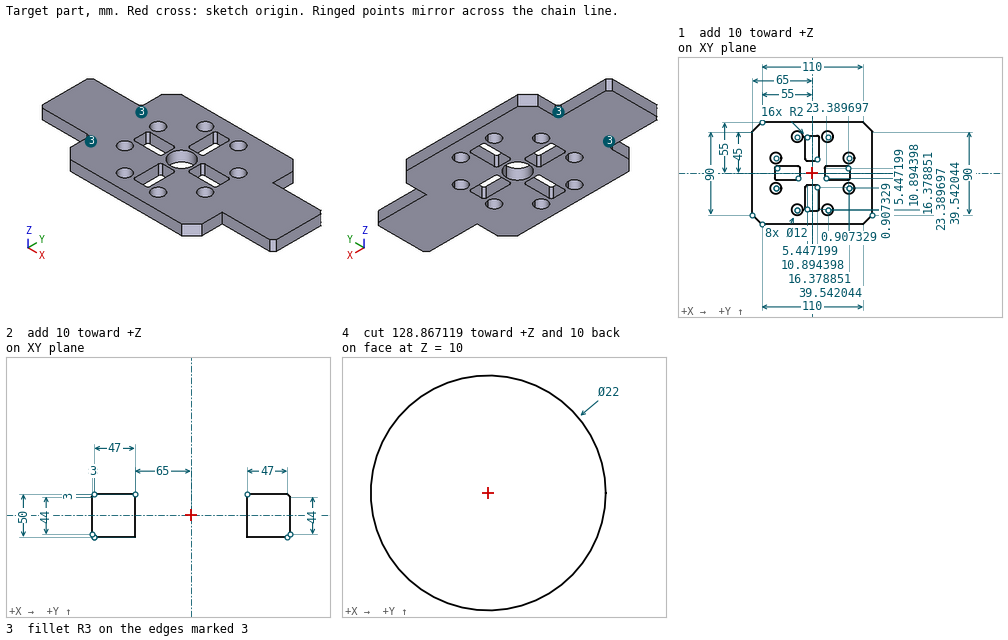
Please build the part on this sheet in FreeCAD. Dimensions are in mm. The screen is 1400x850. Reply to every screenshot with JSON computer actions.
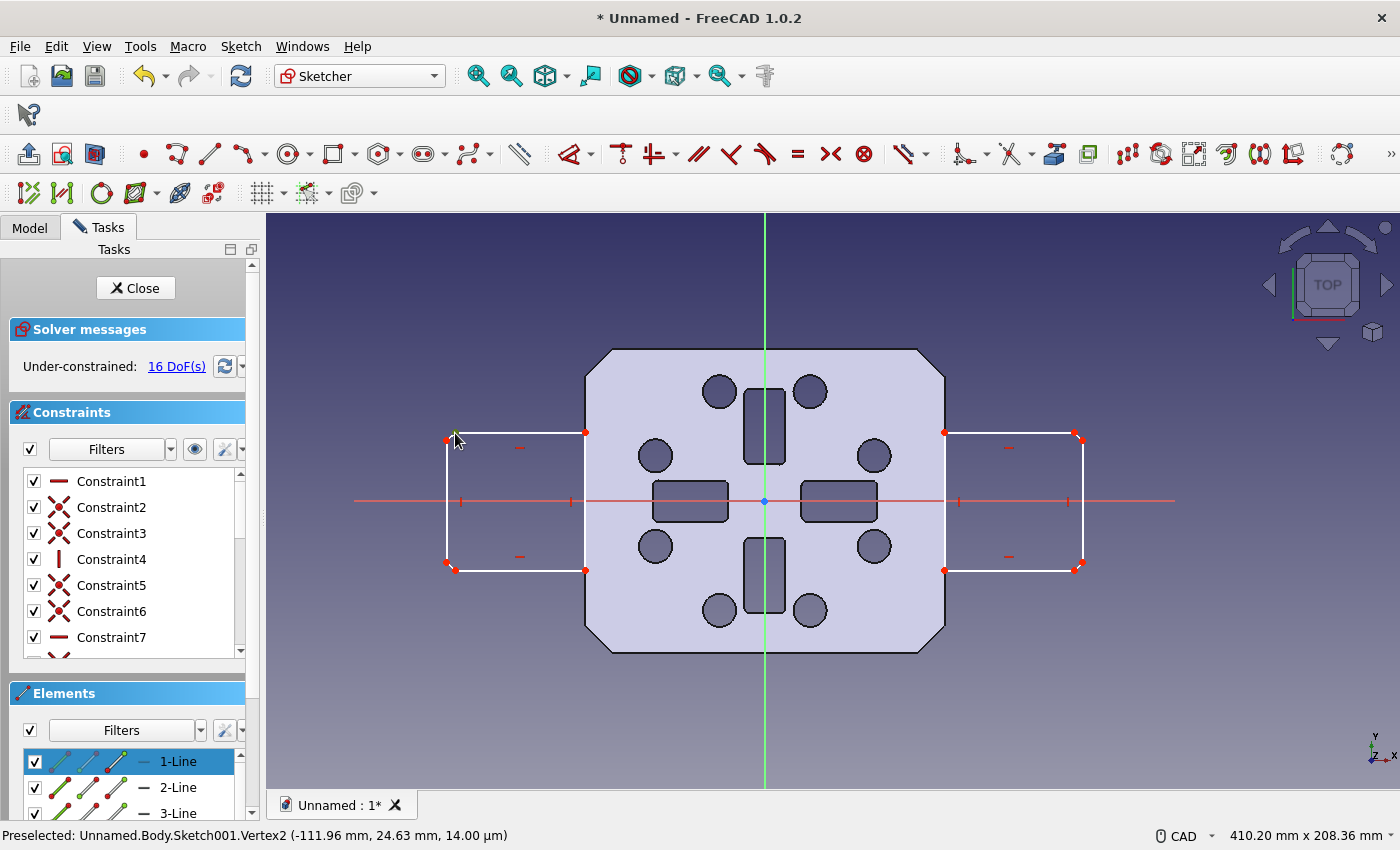
{"action": "left_click", "coordinate": [455, 571]}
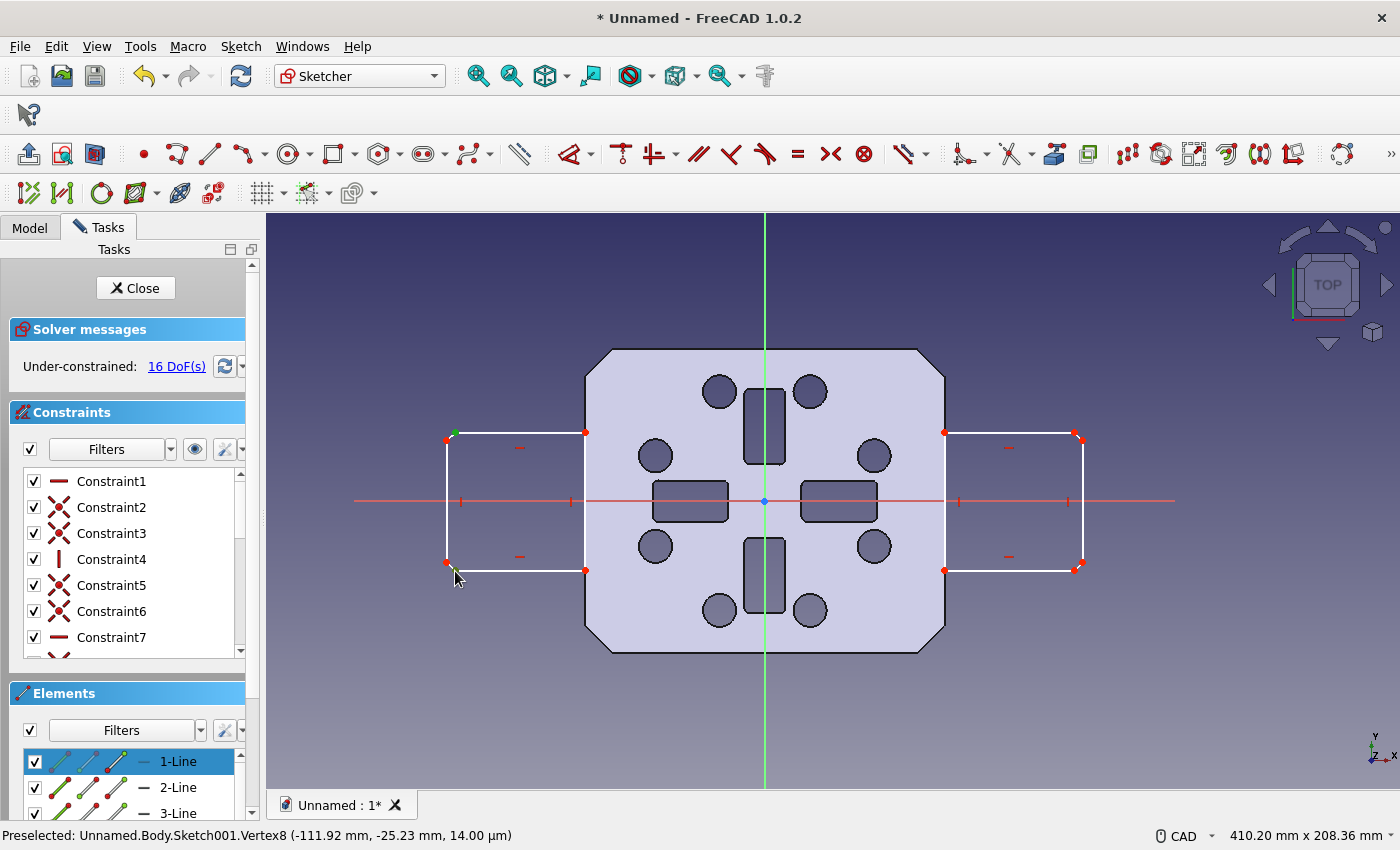
{"action": "left_click", "coordinate": [361, 501]}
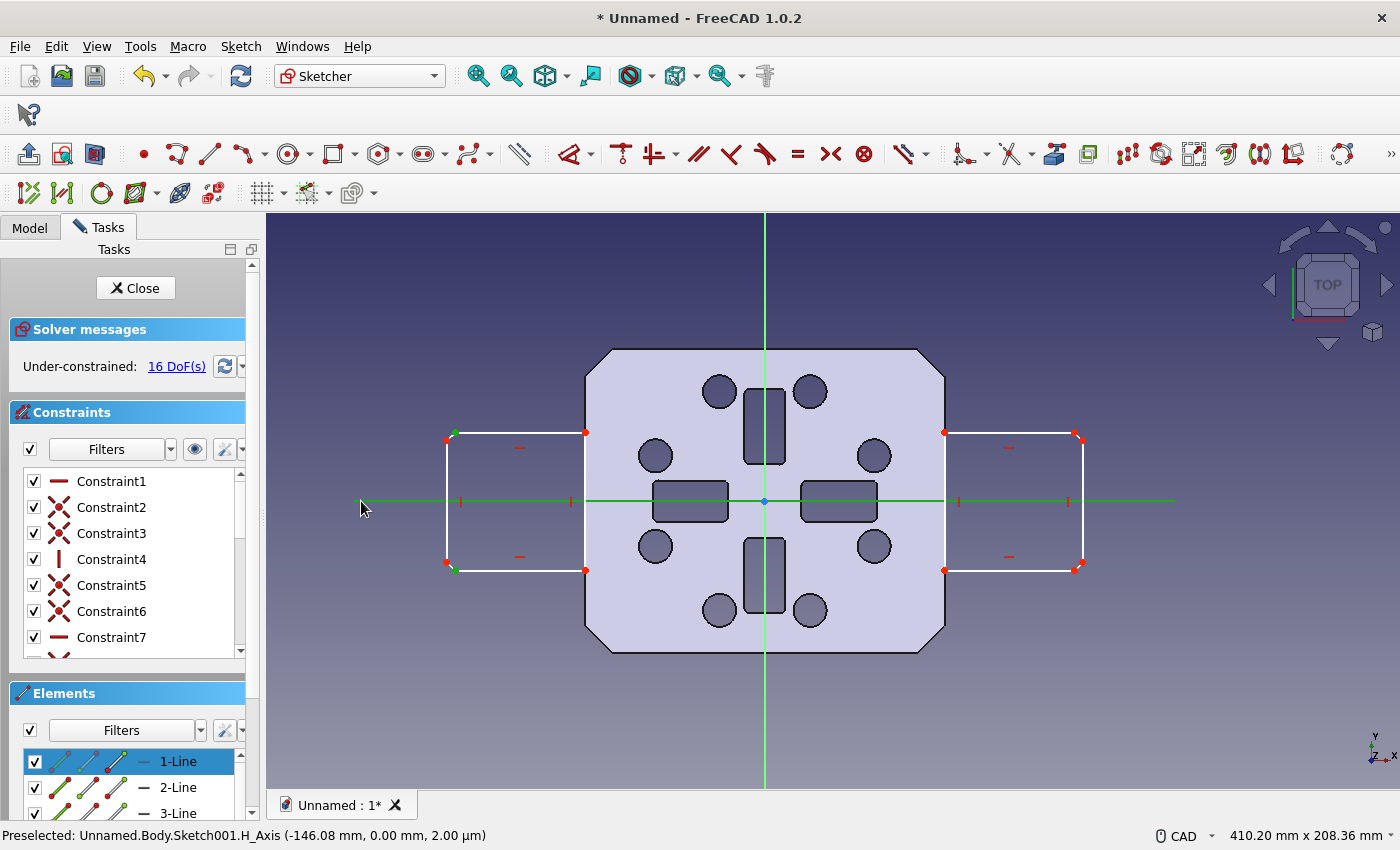
{"action": "left_click", "coordinate": [831, 154]}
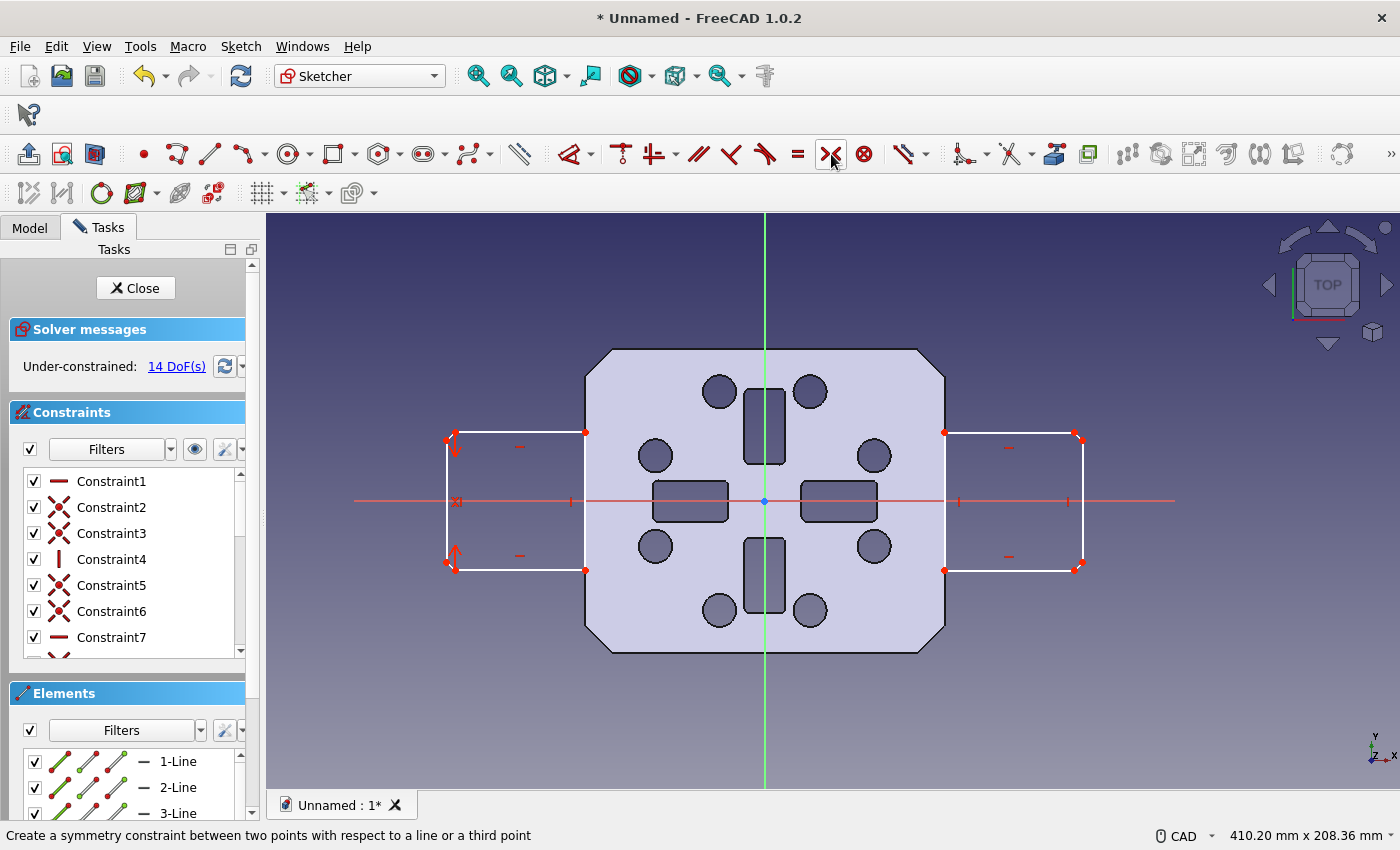
{"action": "left_click", "coordinate": [585, 432]}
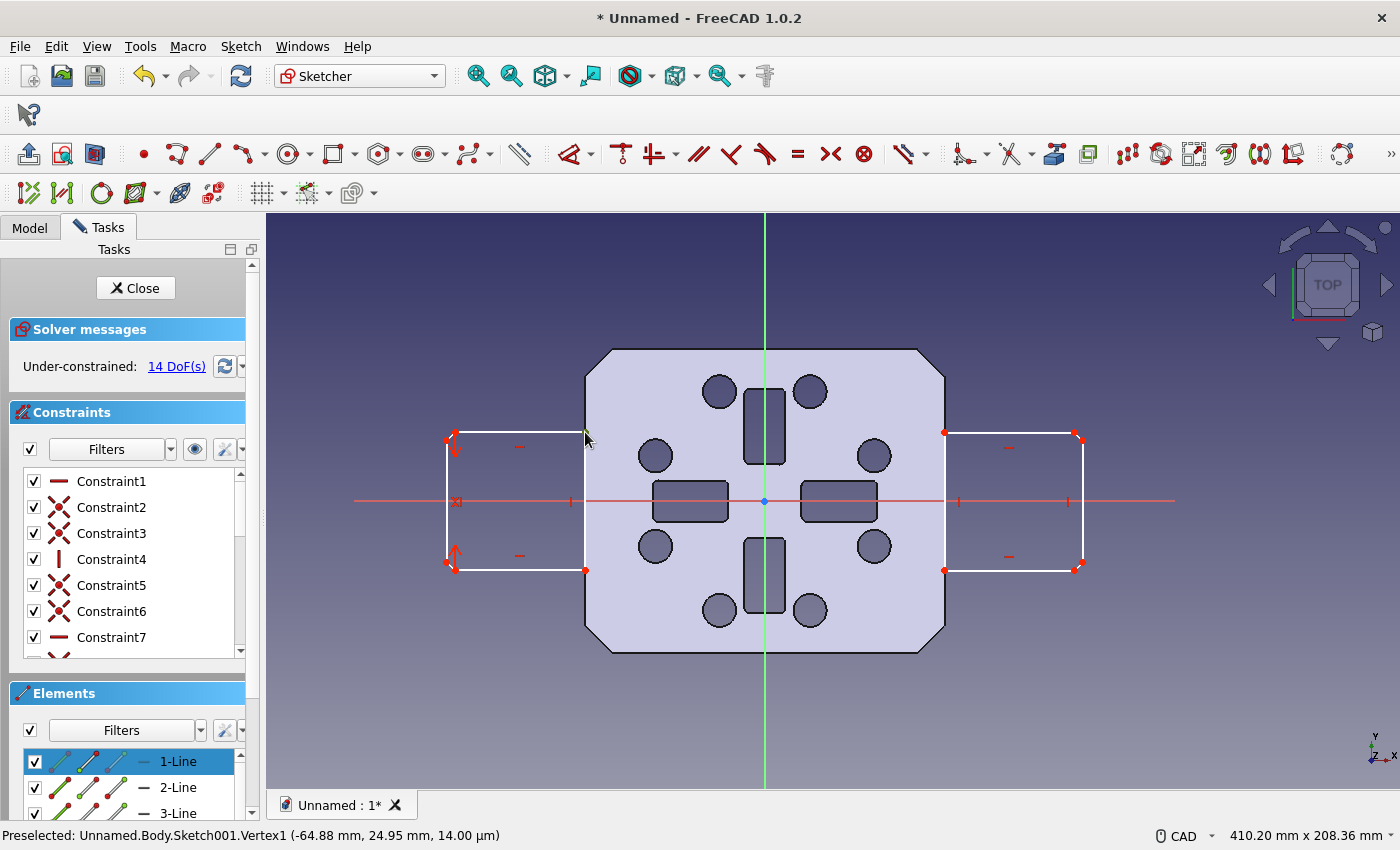
{"action": "left_click", "coordinate": [945, 433]}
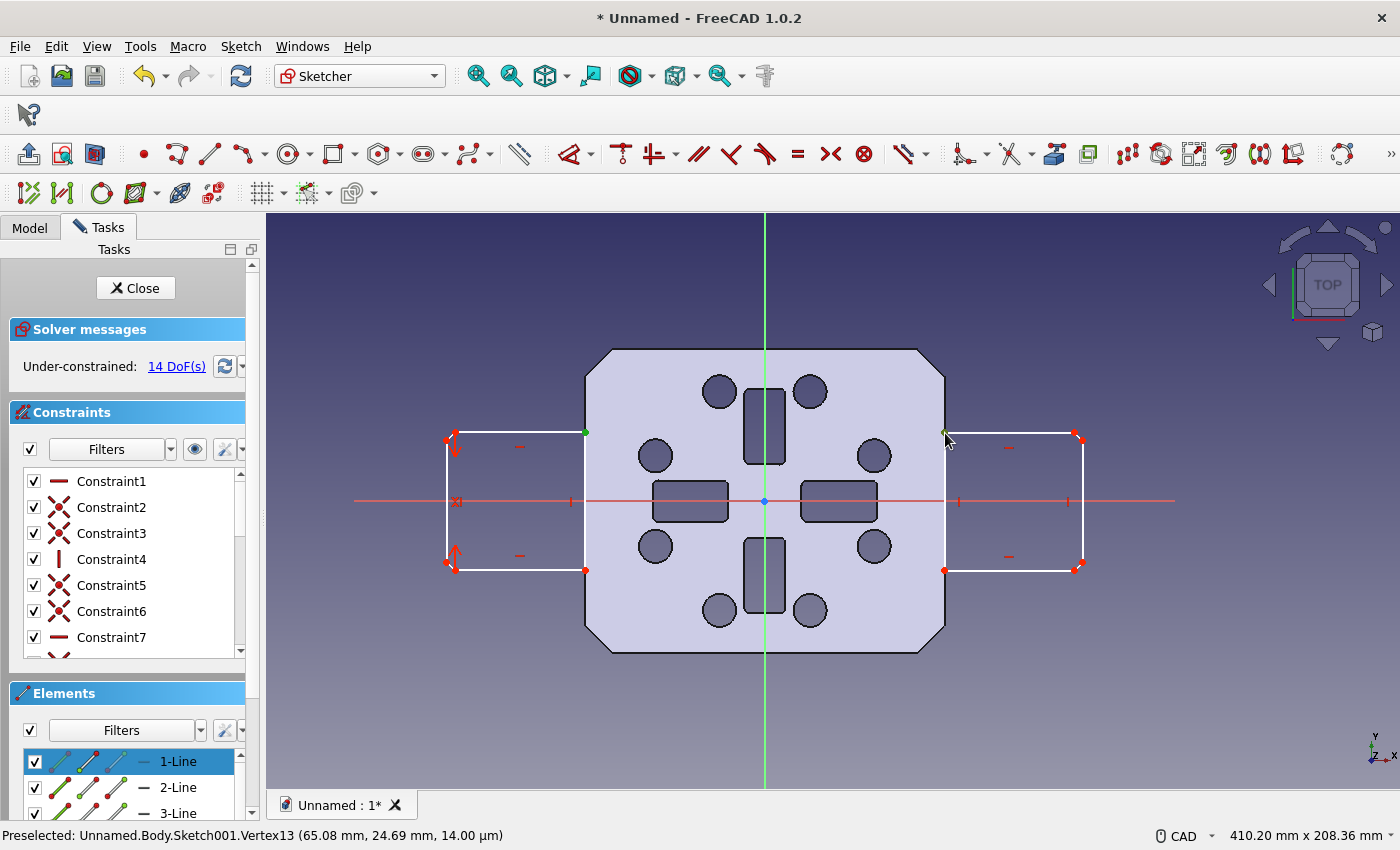
{"action": "left_click", "coordinate": [765, 724]}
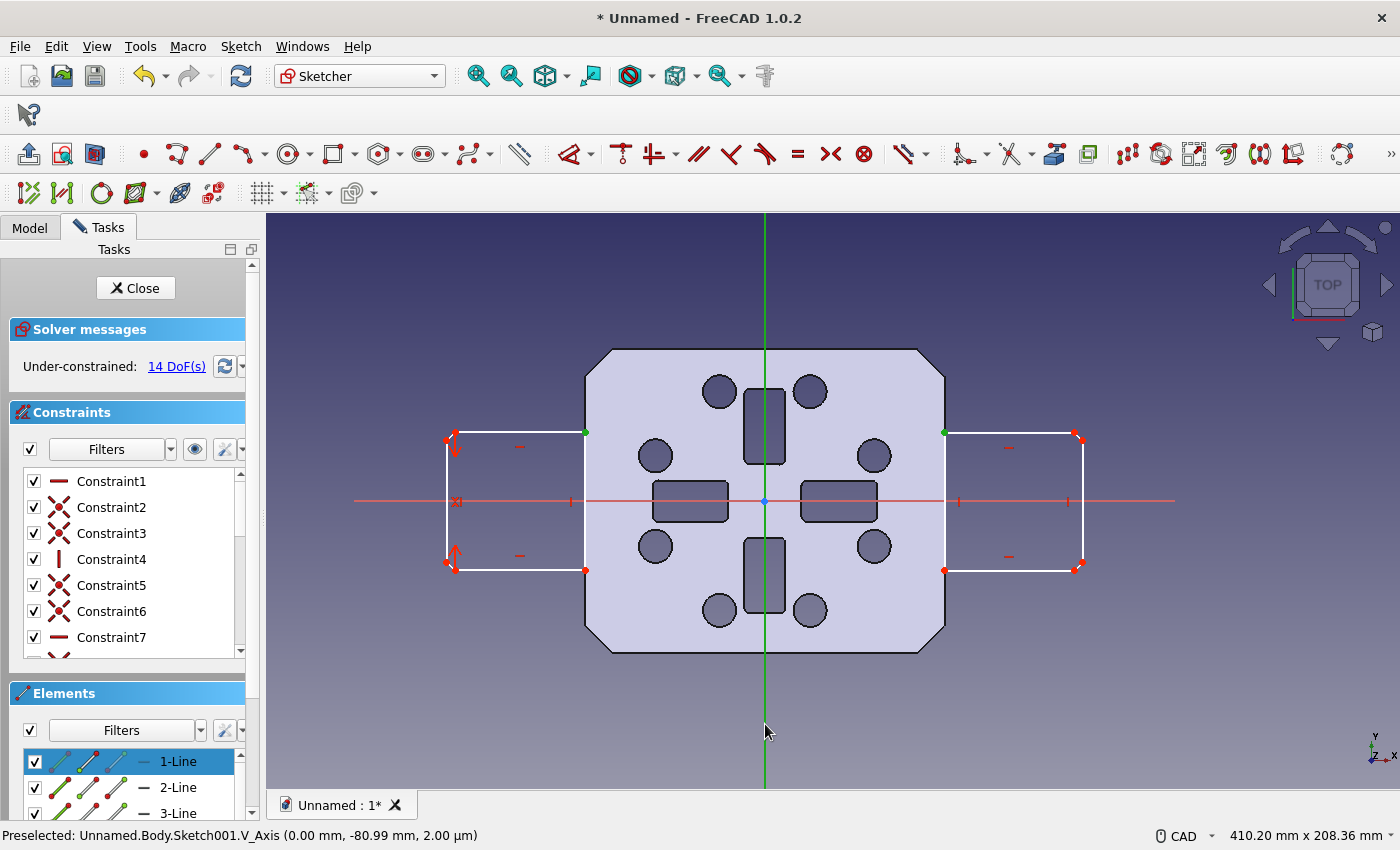
{"action": "left_click", "coordinate": [831, 154]}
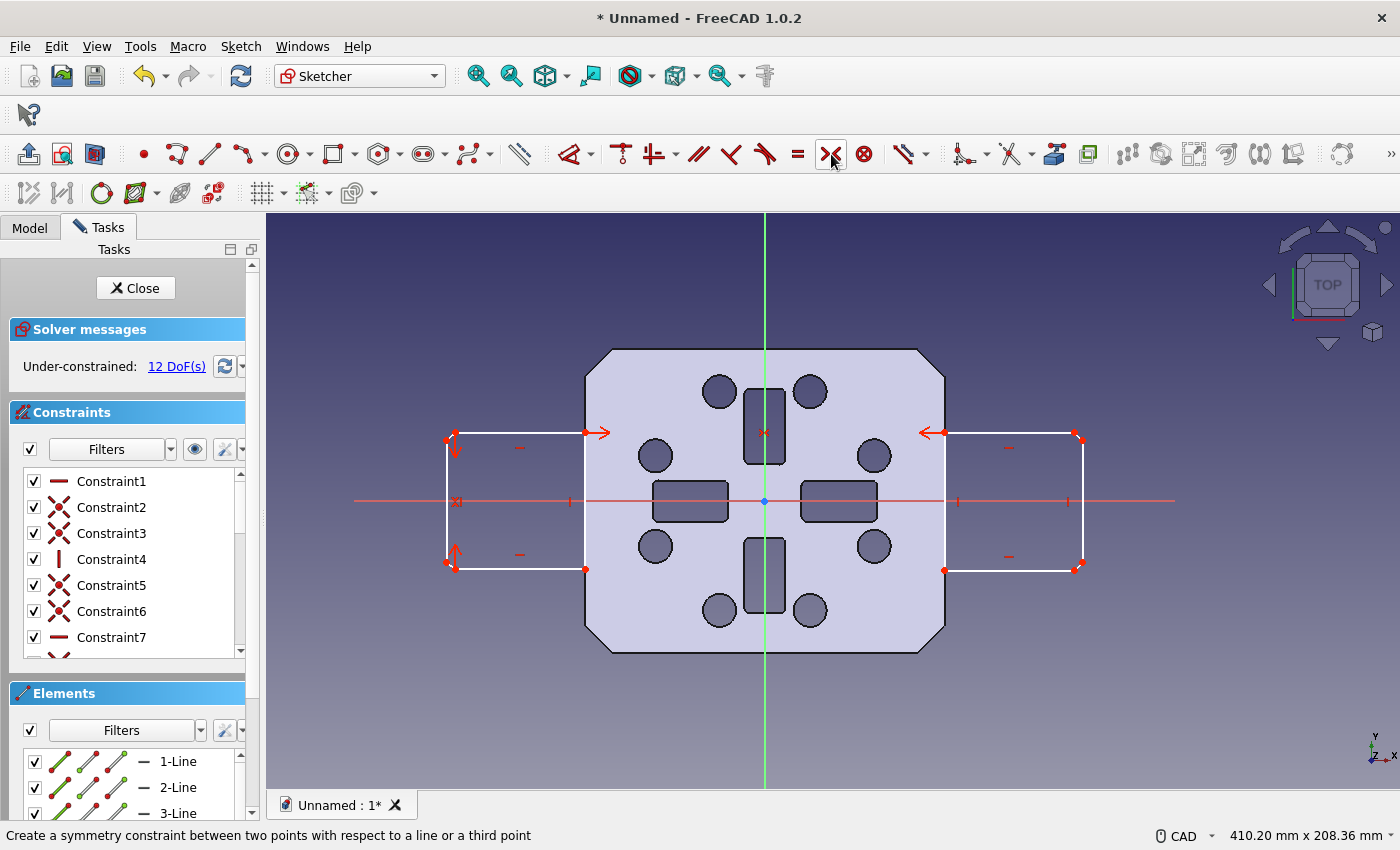
{"action": "left_click", "coordinate": [455, 569]}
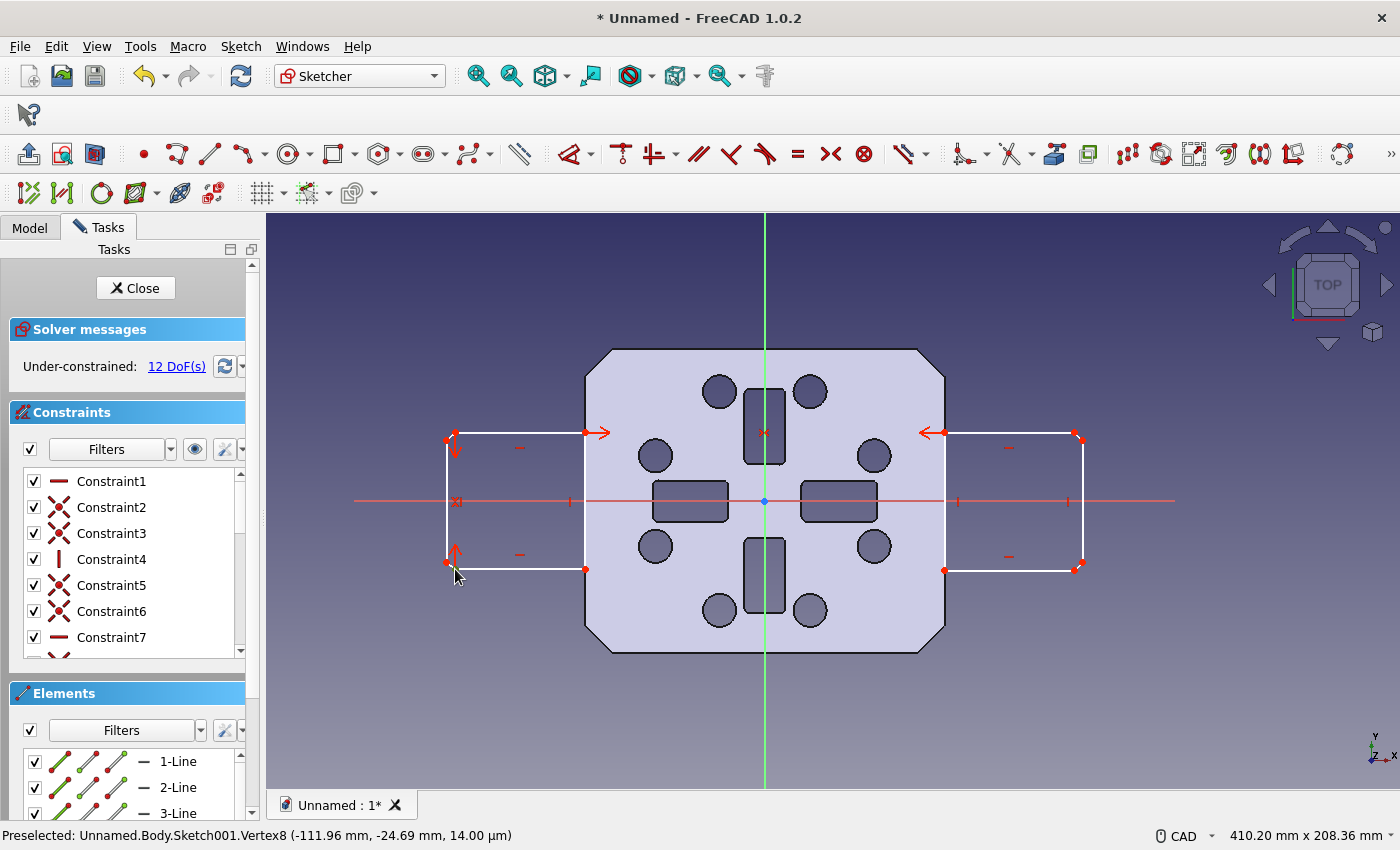
{"action": "left_click", "coordinate": [1074, 571]}